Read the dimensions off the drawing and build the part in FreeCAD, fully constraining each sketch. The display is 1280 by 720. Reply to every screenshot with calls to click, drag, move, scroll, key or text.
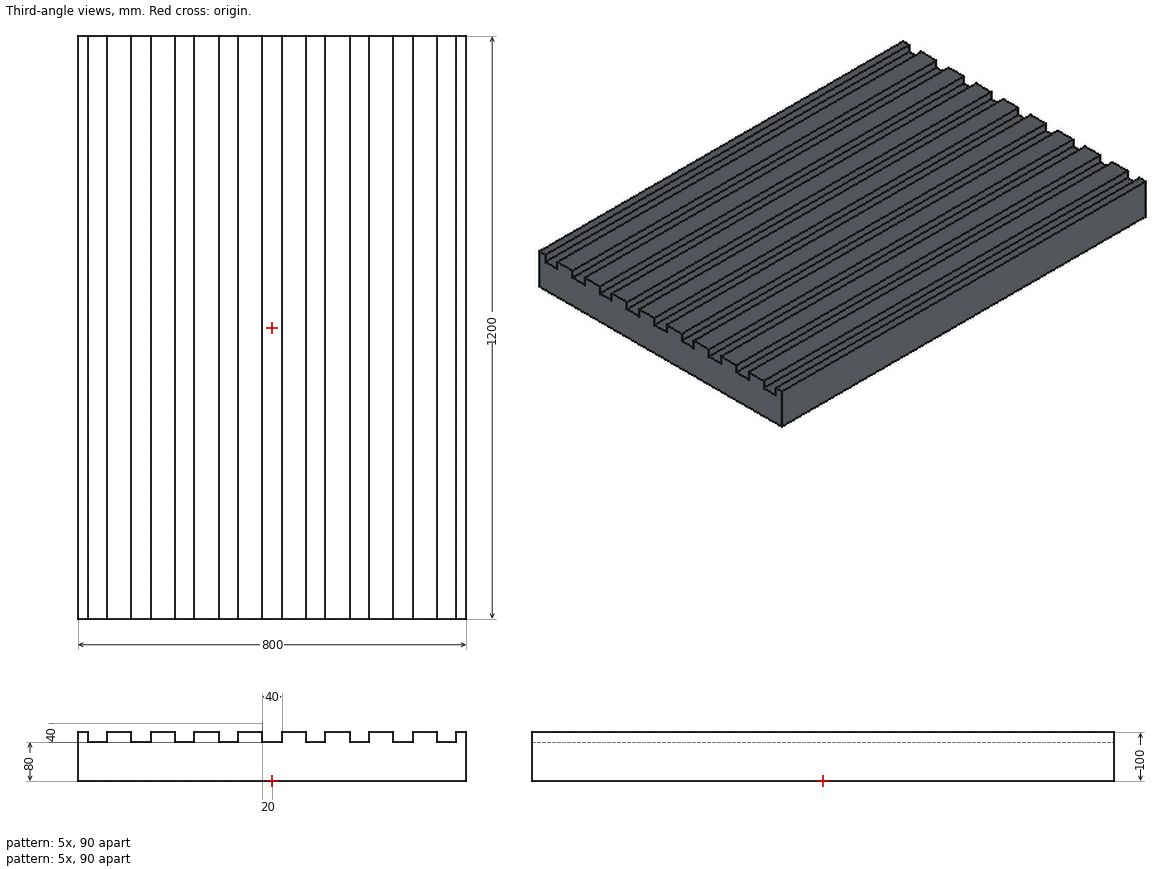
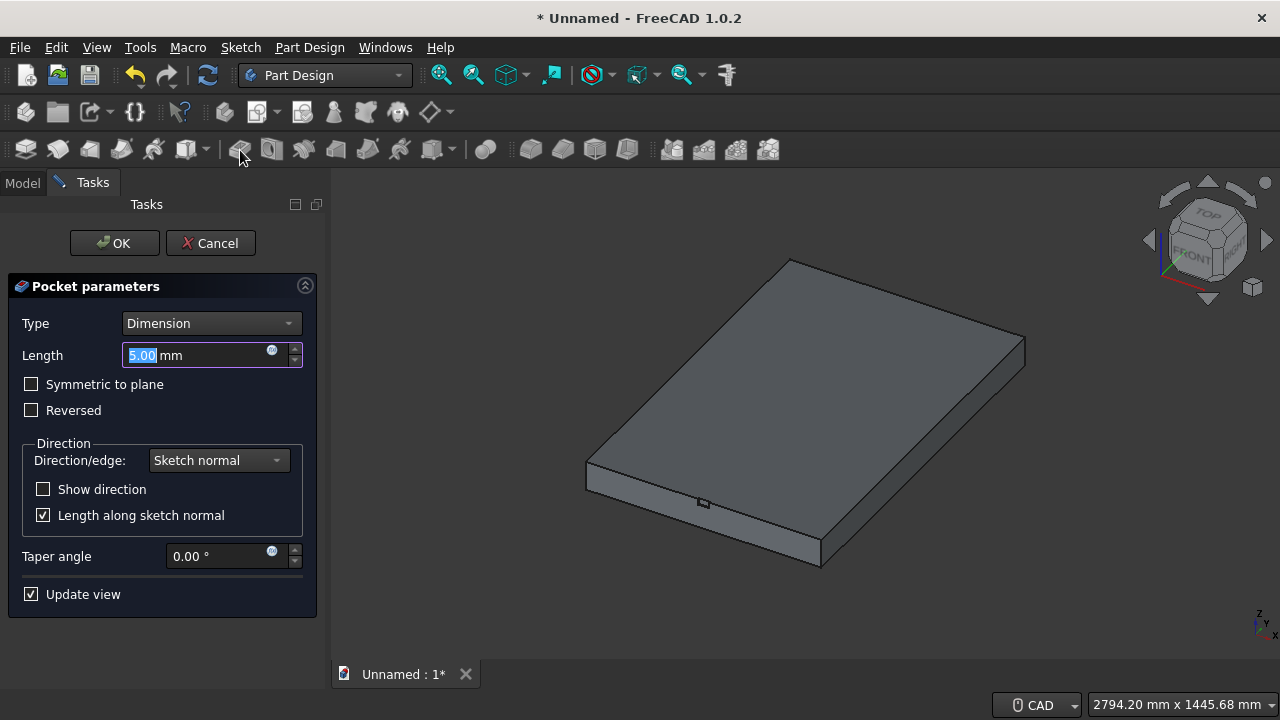
click(212, 324)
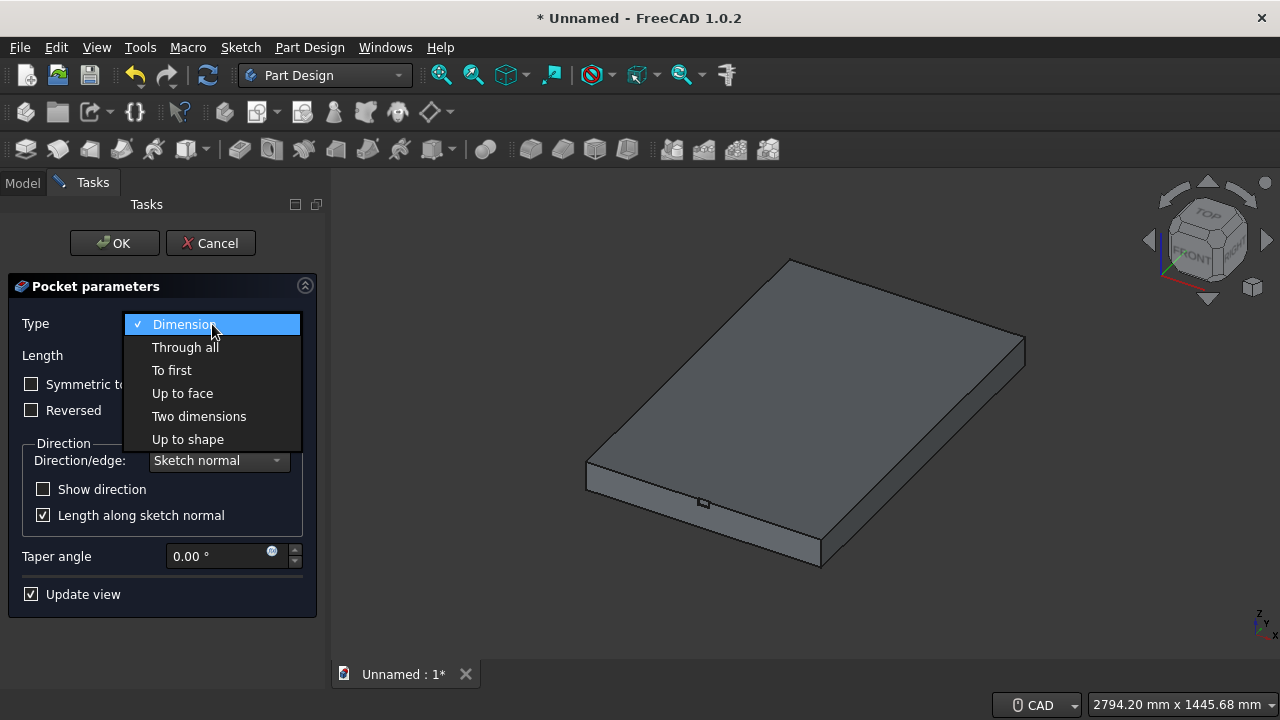
click(212, 348)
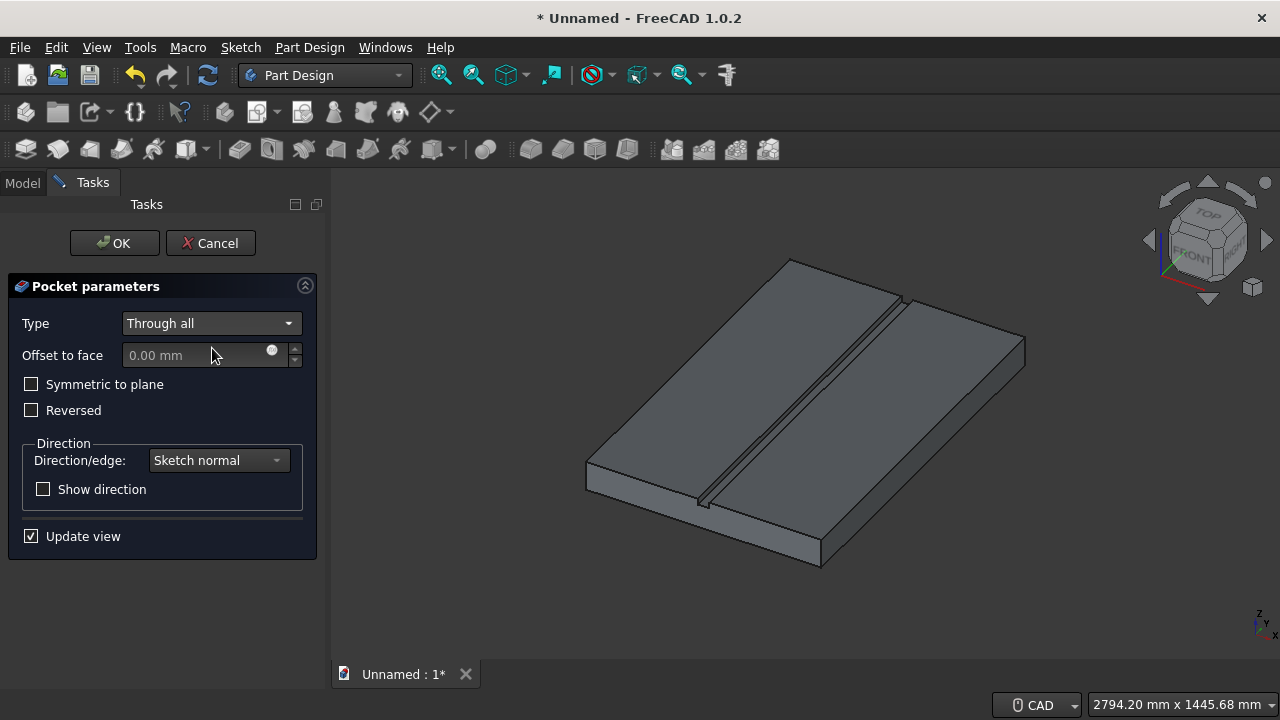
click(115, 243)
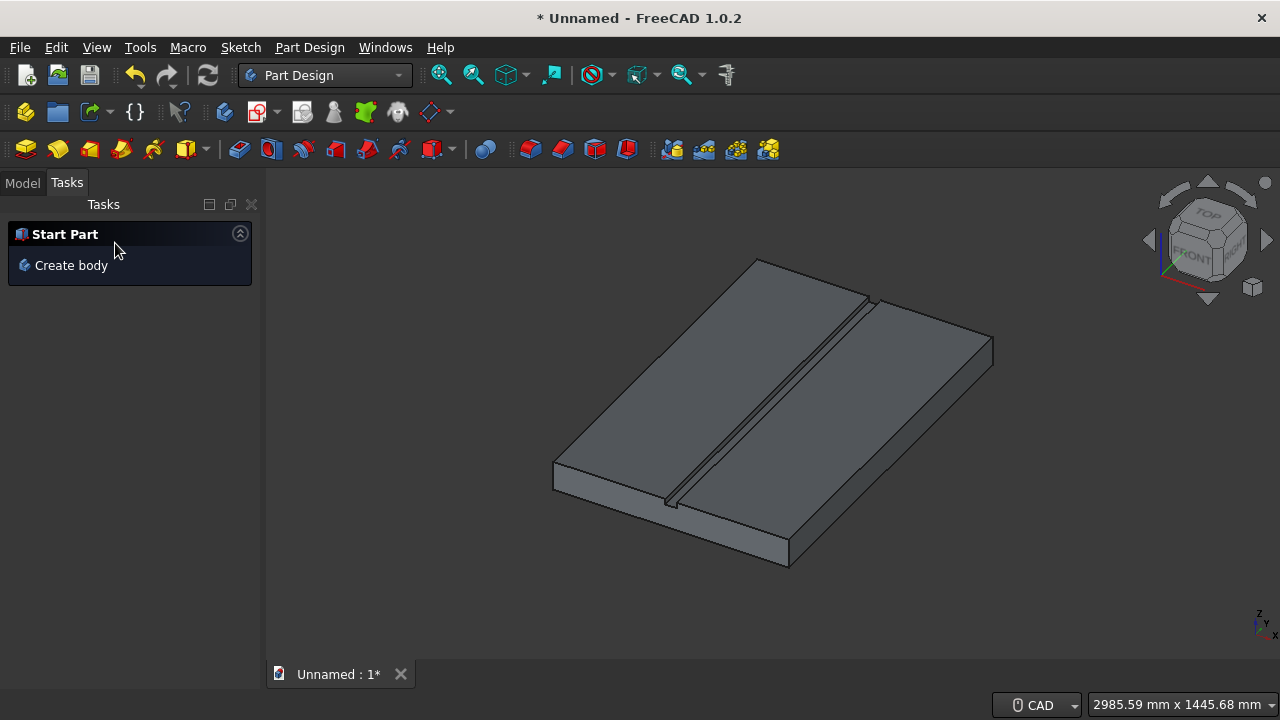
click(23, 182)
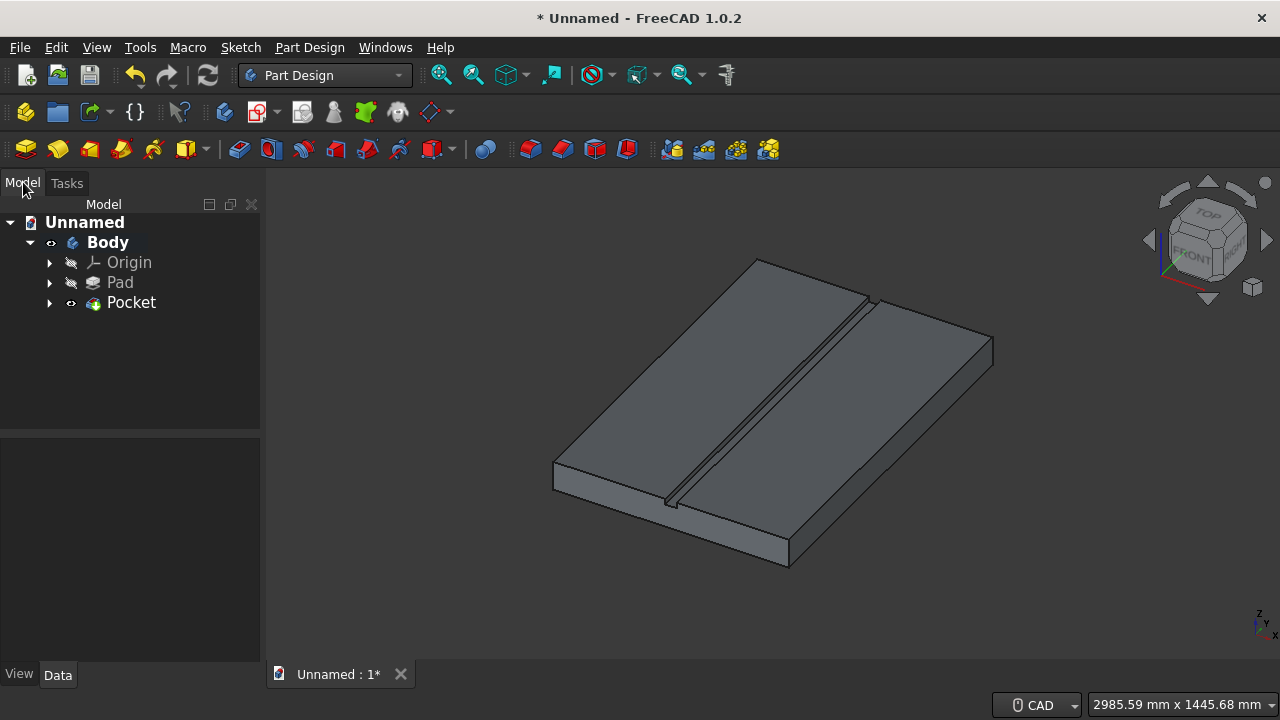
click(116, 303)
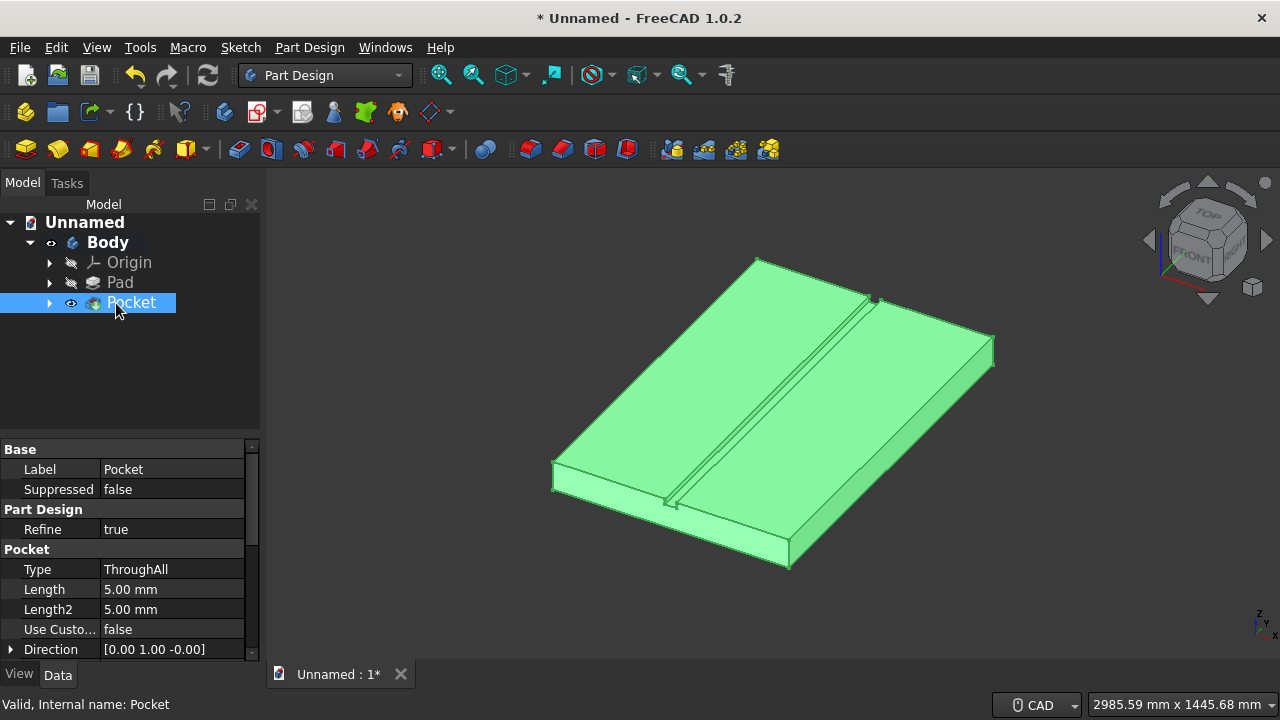
click(704, 150)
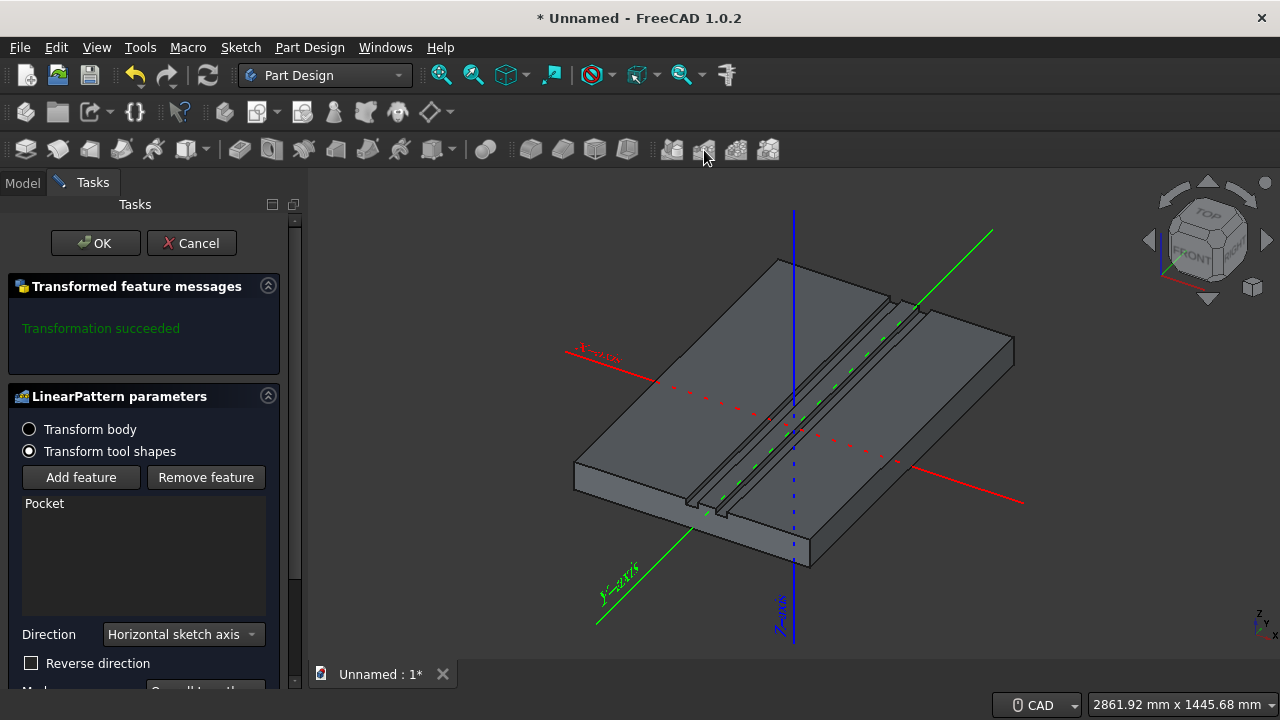
click(184, 634)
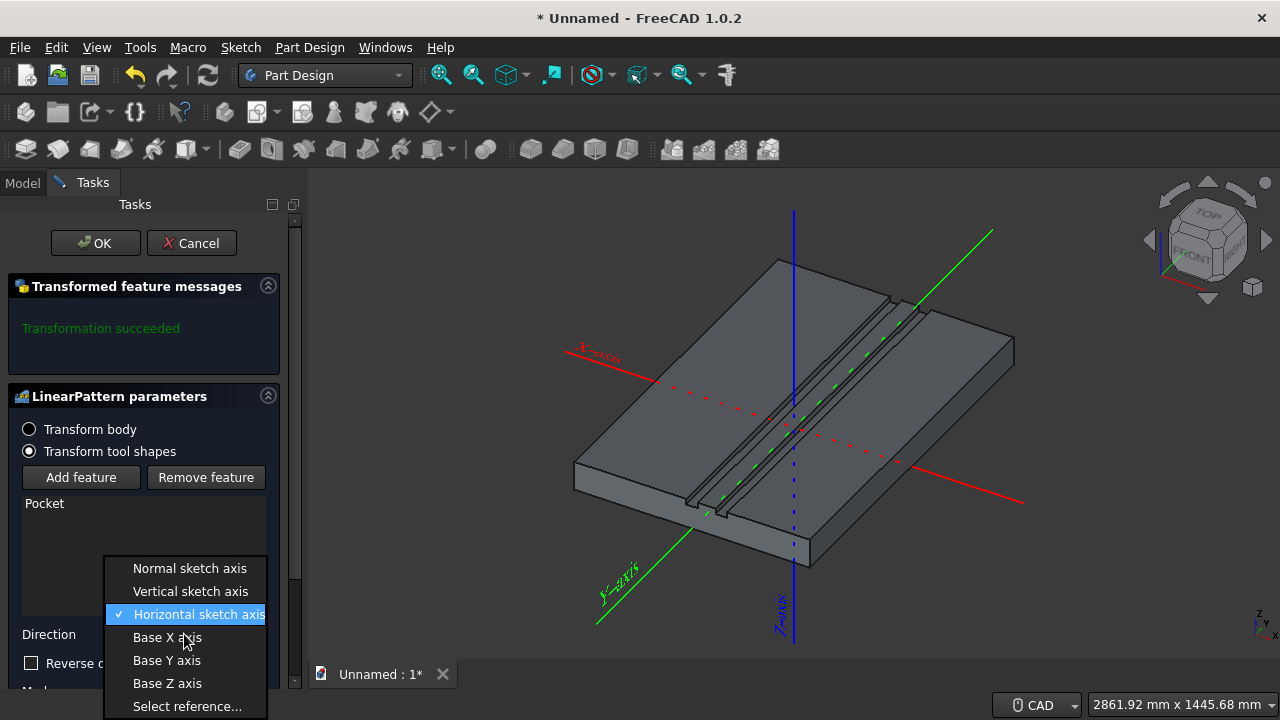
click(184, 638)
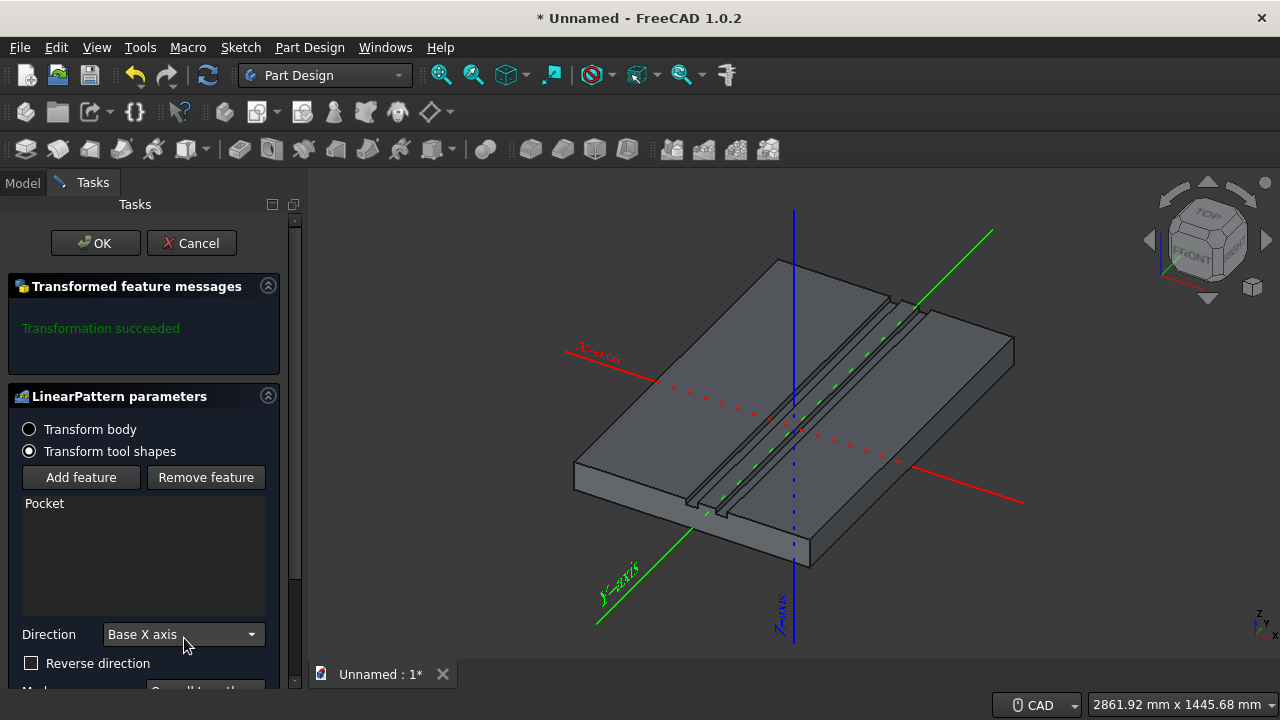
scroll(295, 451, down, 2)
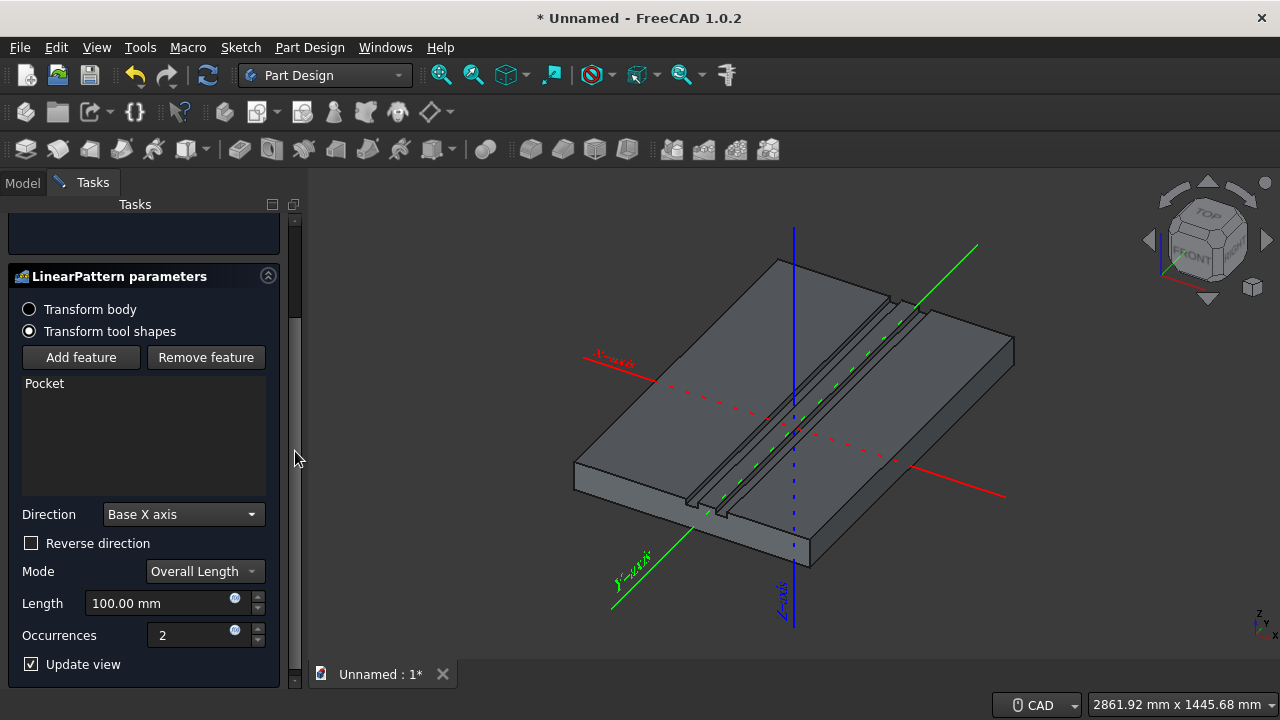
click(206, 572)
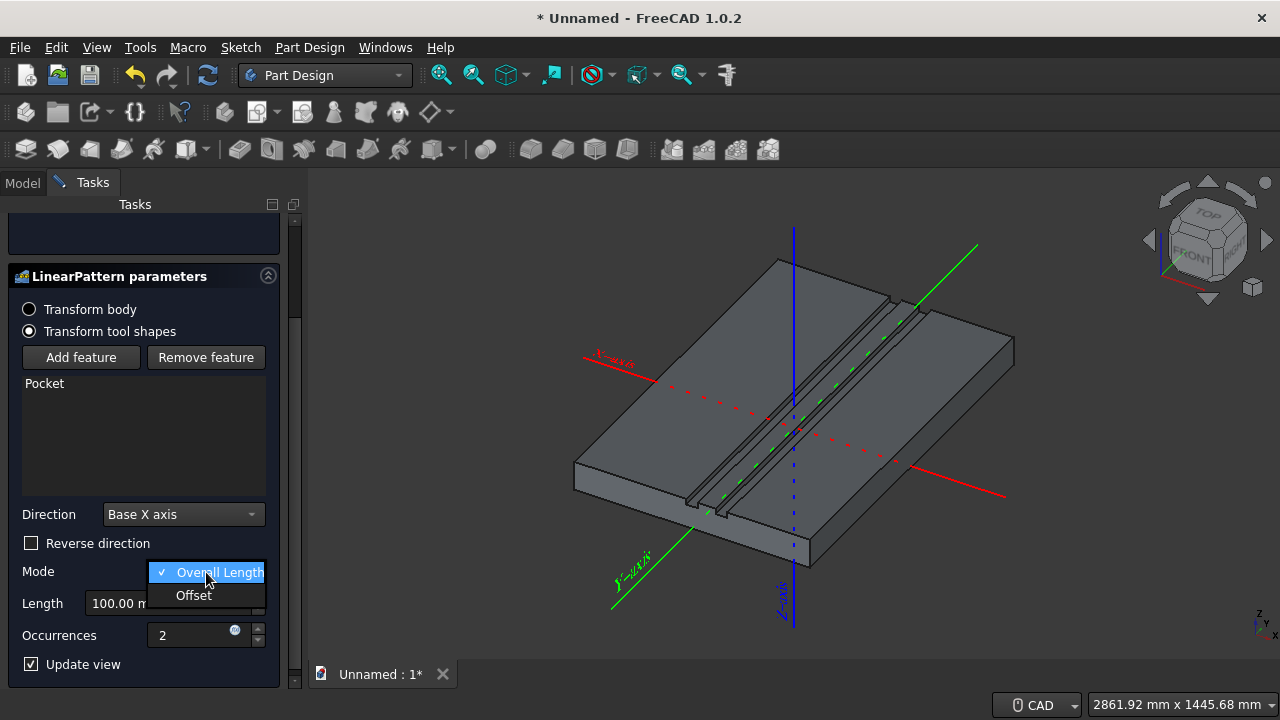
click(206, 596)